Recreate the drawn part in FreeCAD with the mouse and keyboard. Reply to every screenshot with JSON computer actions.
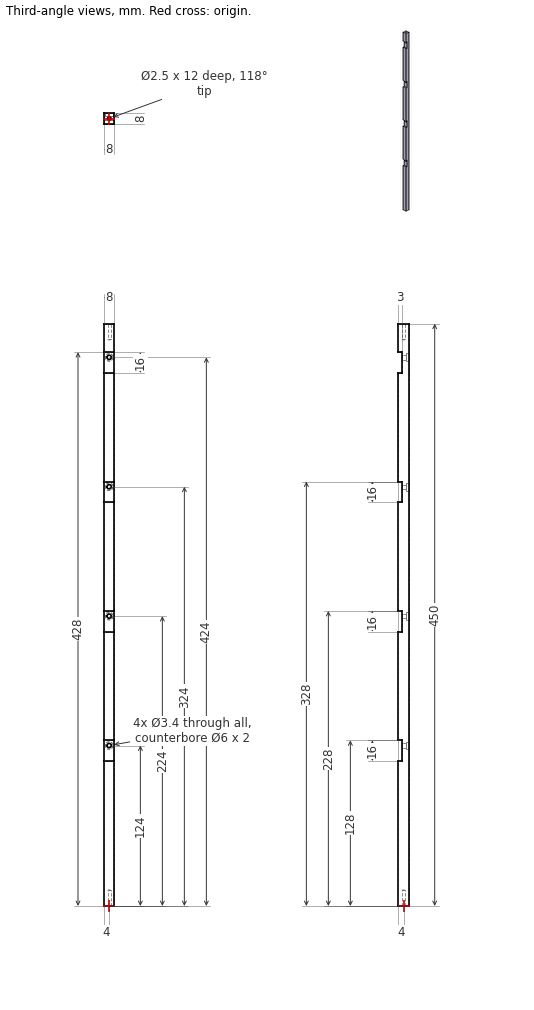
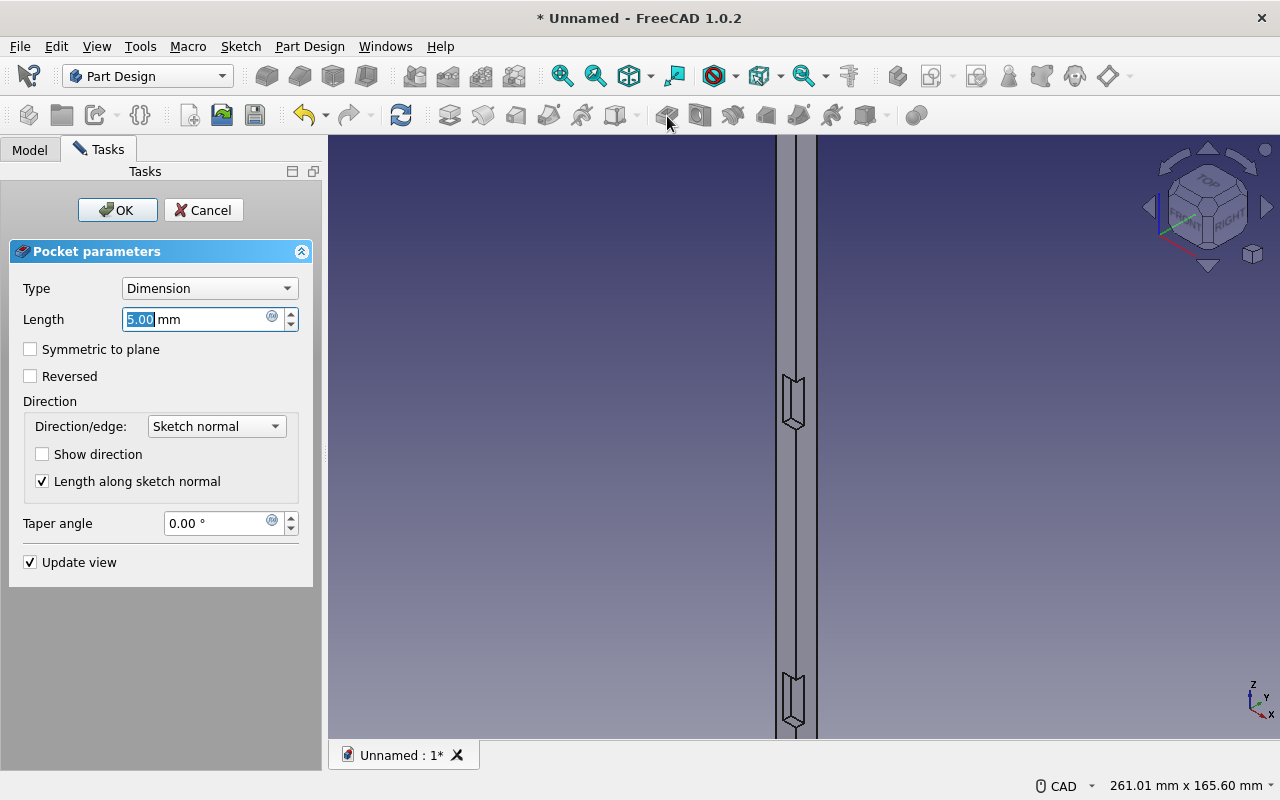
{"action": "left_click", "coordinate": [210, 288]}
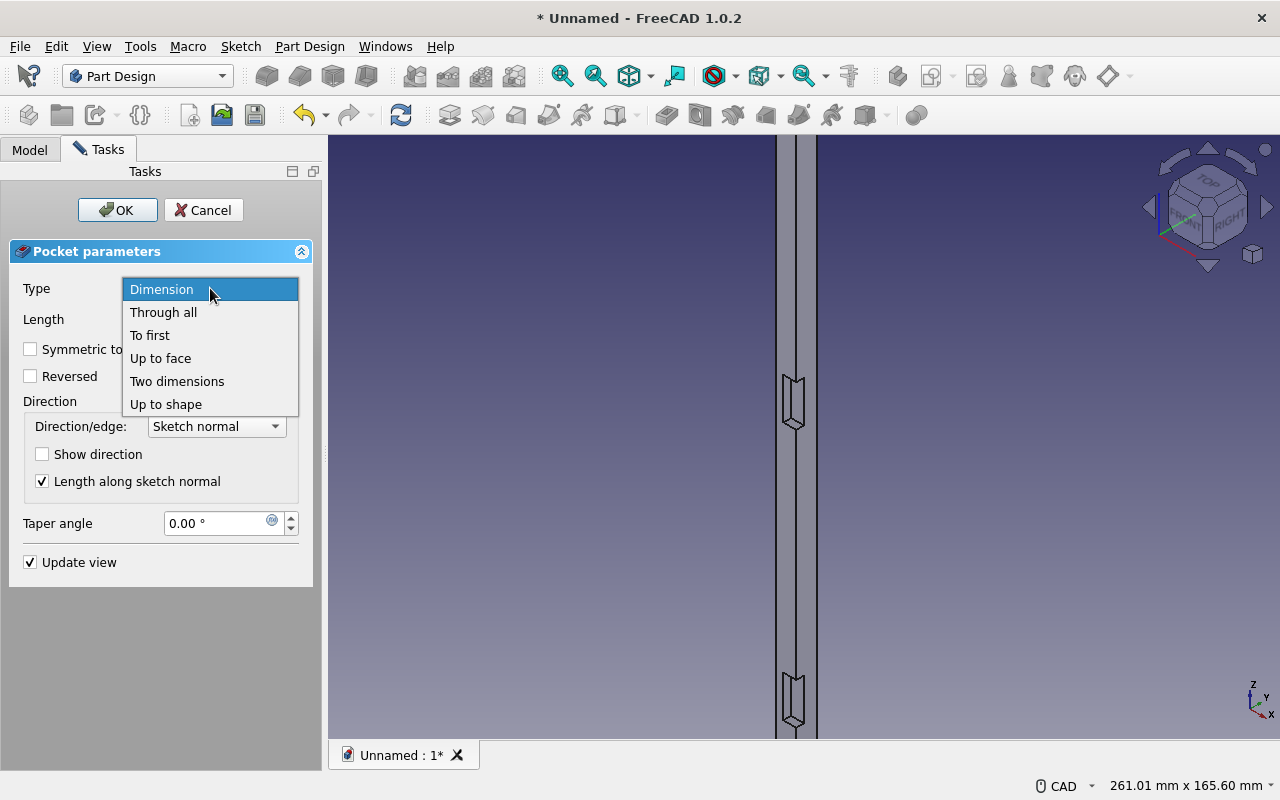
{"action": "left_click", "coordinate": [208, 312]}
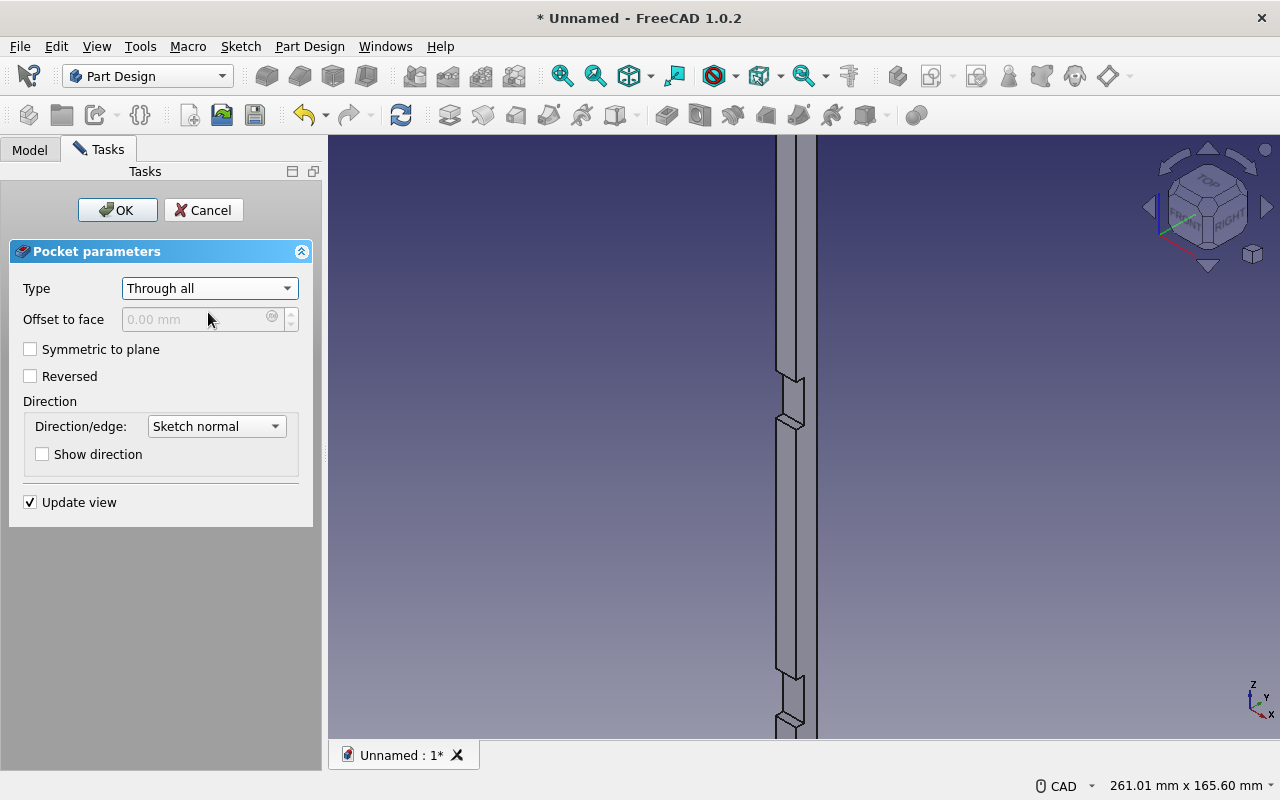
{"action": "left_click", "coordinate": [118, 210]}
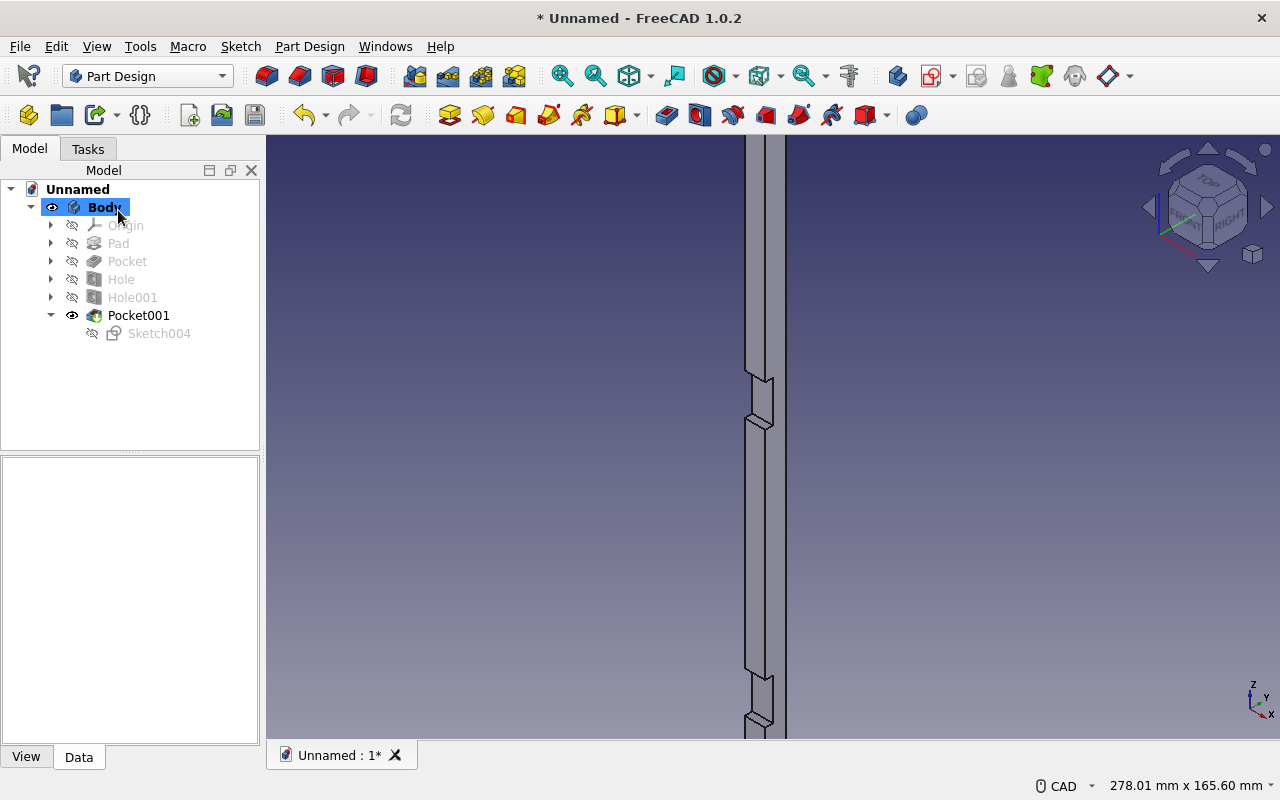
{"action": "key", "text": "v f"}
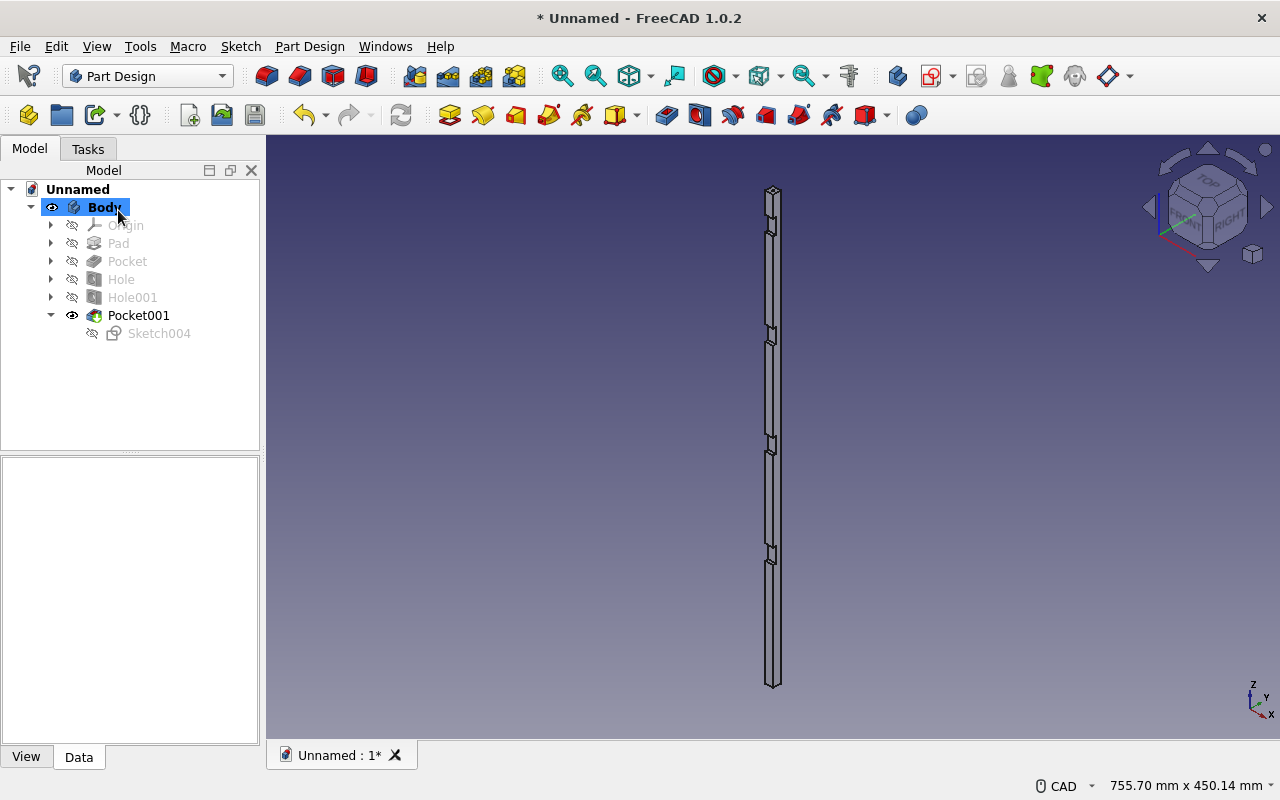
{"action": "key", "text": "4"}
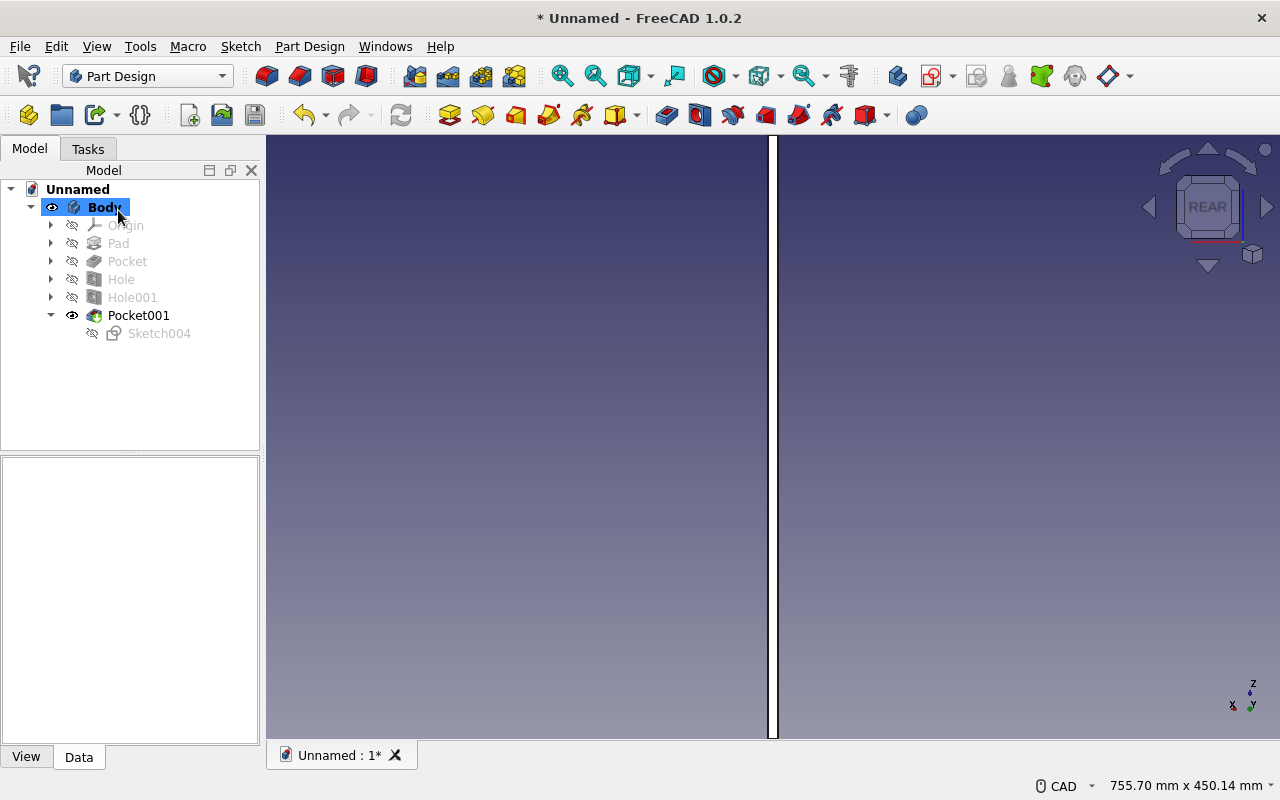
{"action": "key", "text": "v f"}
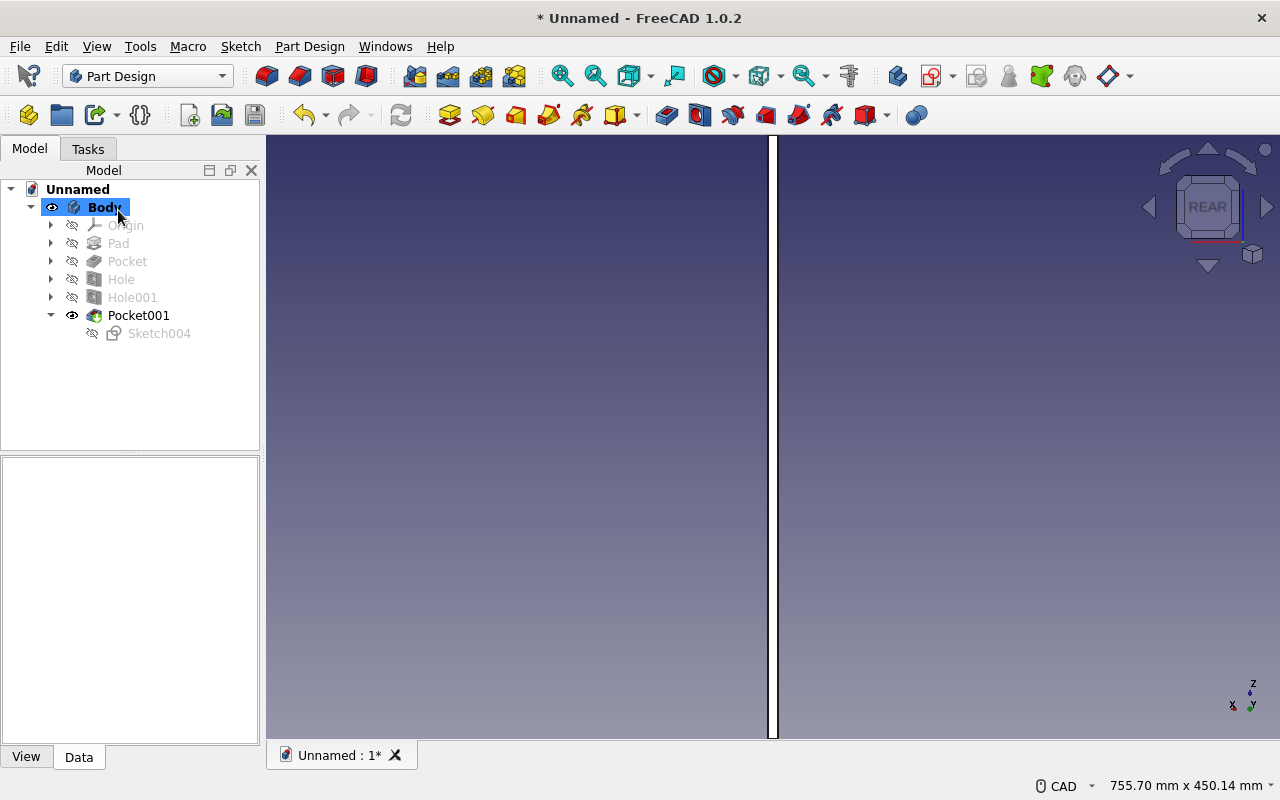
{"action": "scroll", "coordinate": [773, 177], "scroll_direction": "up", "scroll_amount": 5}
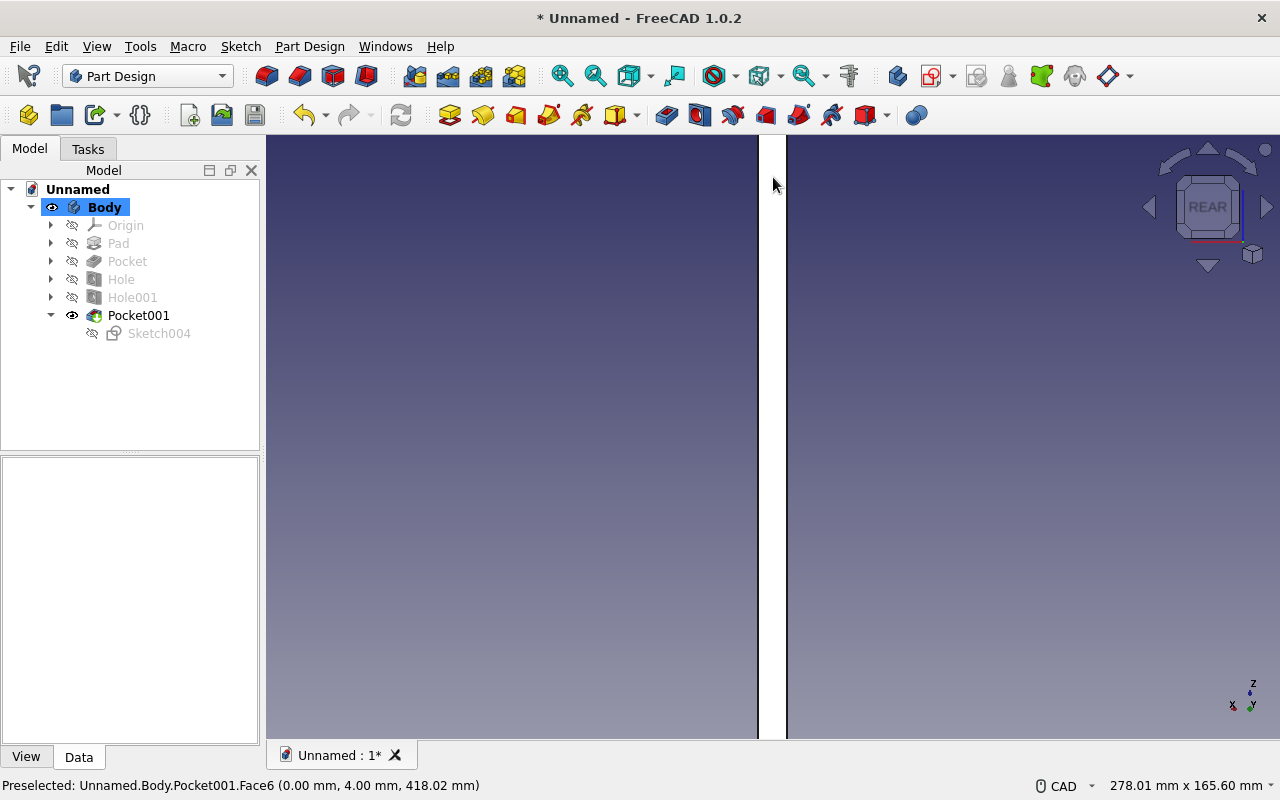
{"action": "left_click", "coordinate": [772, 179]}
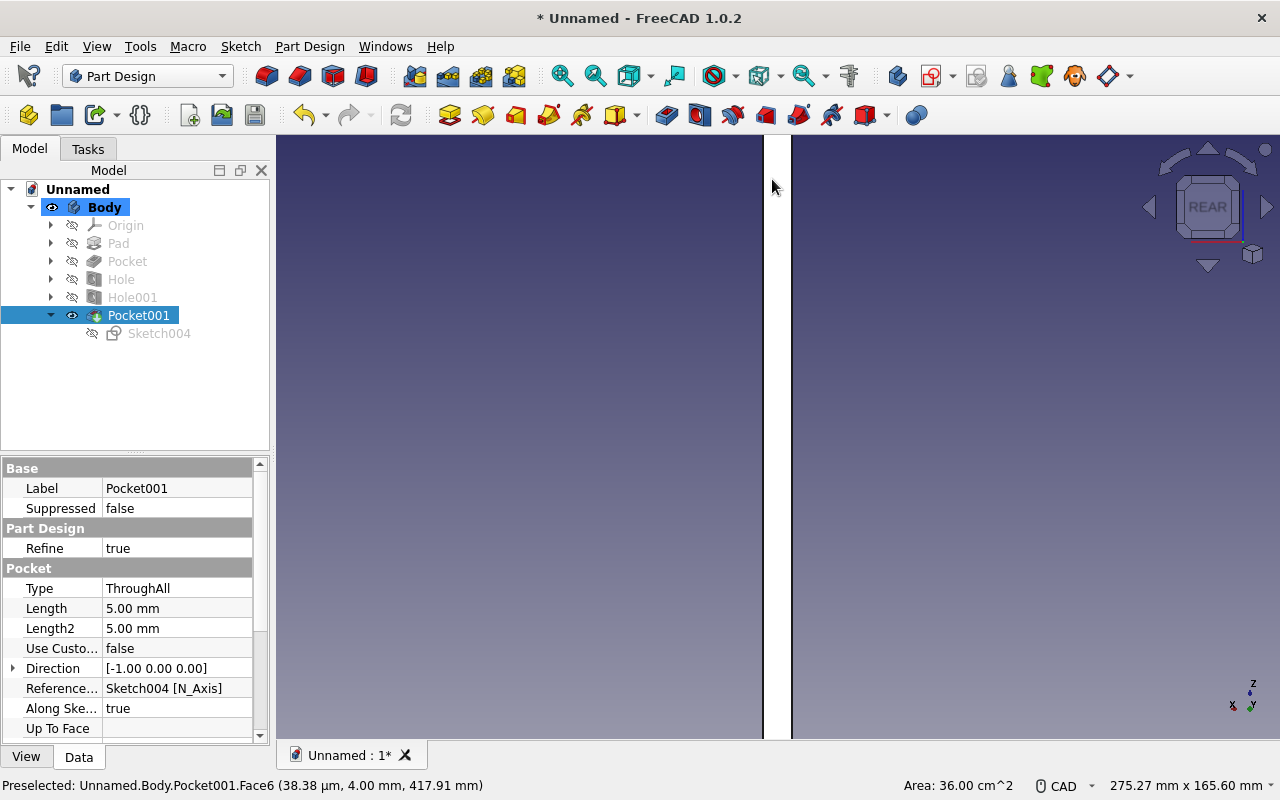
{"action": "left_click", "coordinate": [930, 76]}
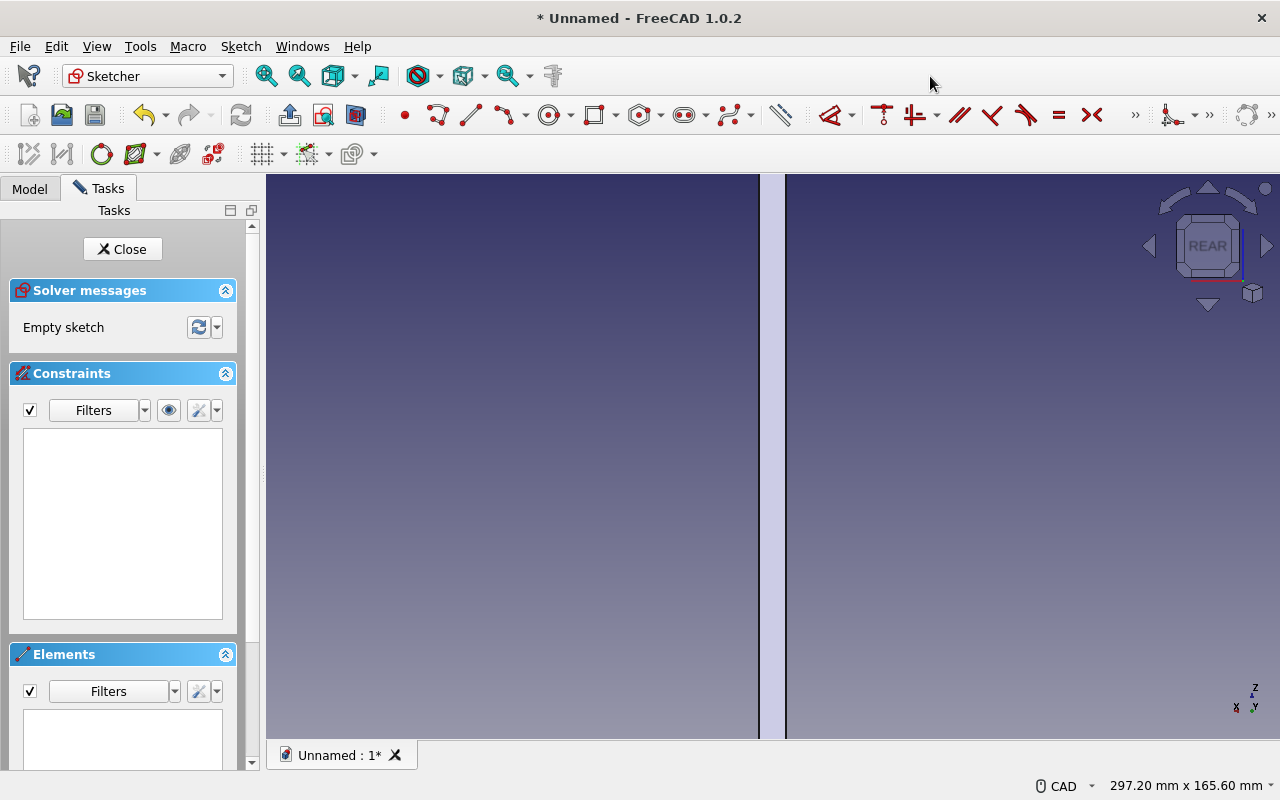
{"action": "scroll", "coordinate": [682, 306], "scroll_direction": "down", "scroll_amount": 7}